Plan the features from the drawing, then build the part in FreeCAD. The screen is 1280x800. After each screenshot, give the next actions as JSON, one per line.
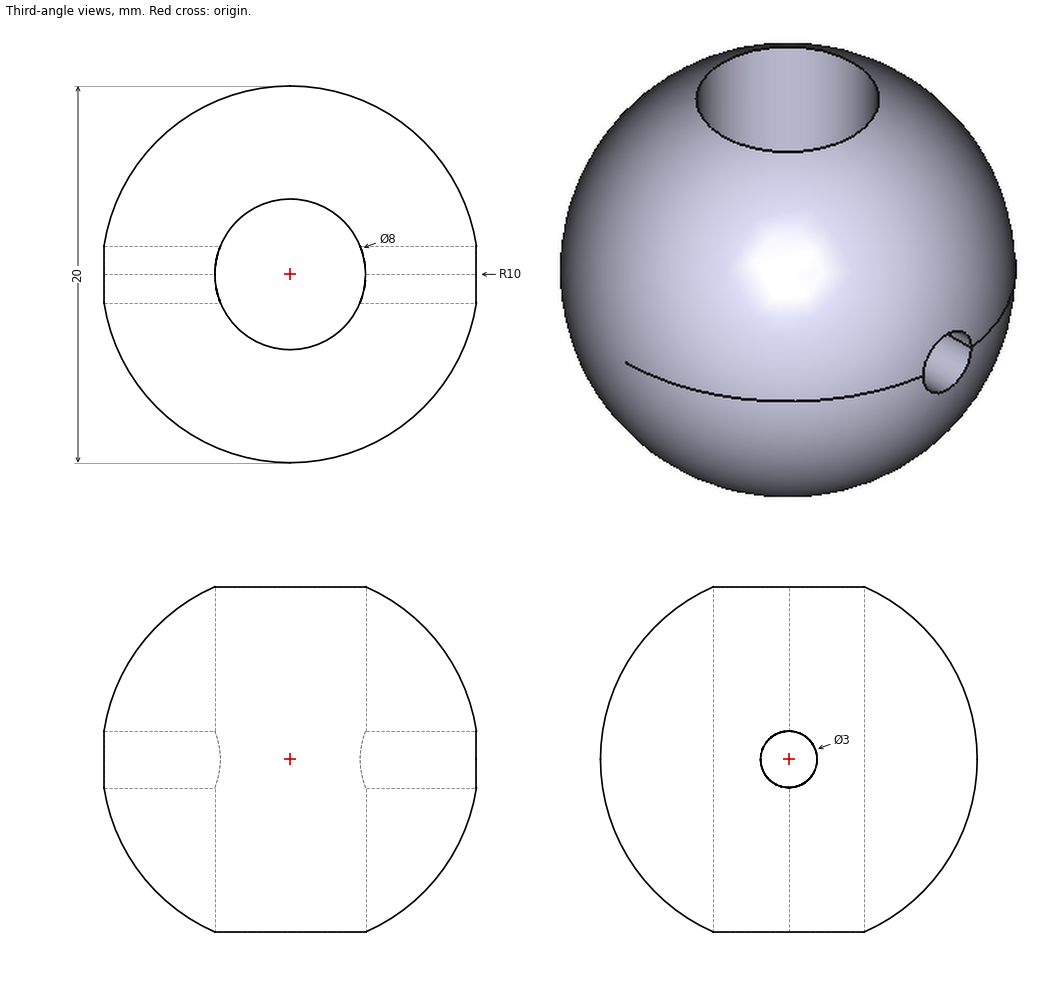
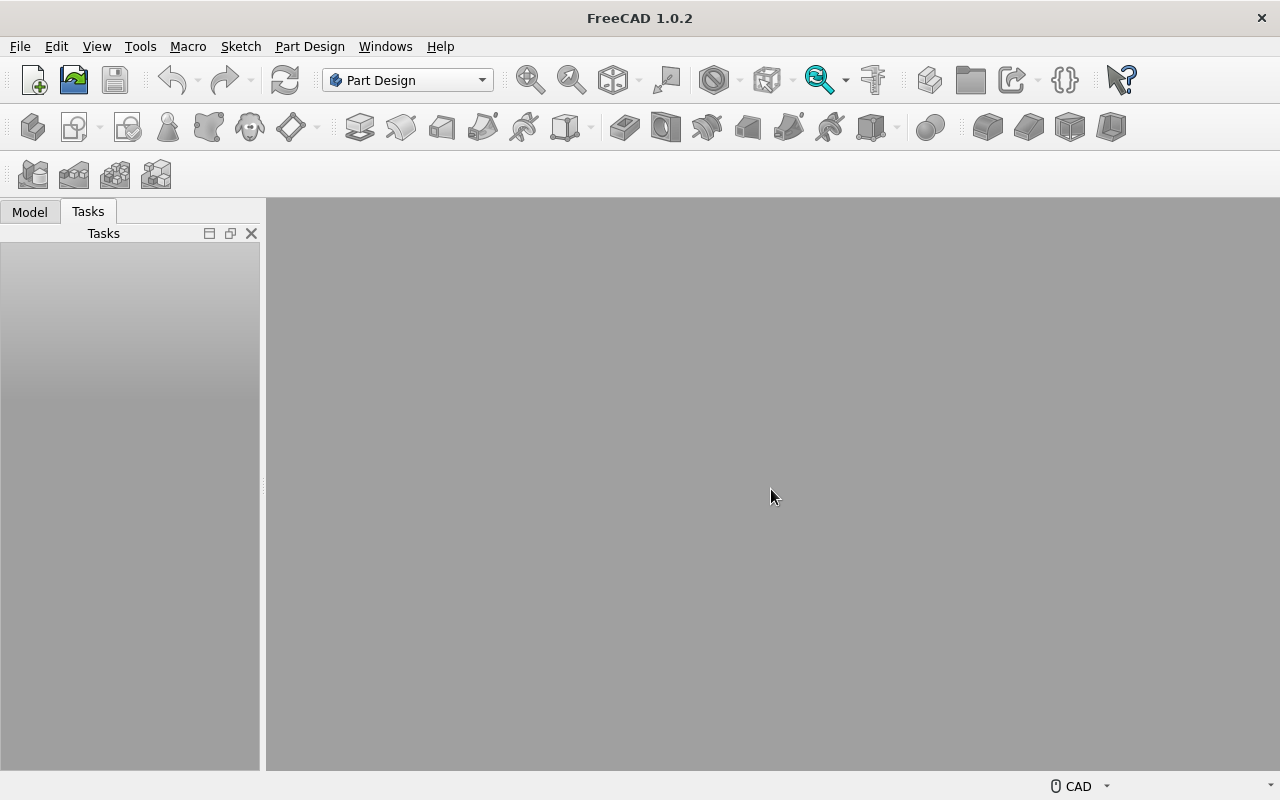
{"action": "left_click", "coordinate": [33, 80]}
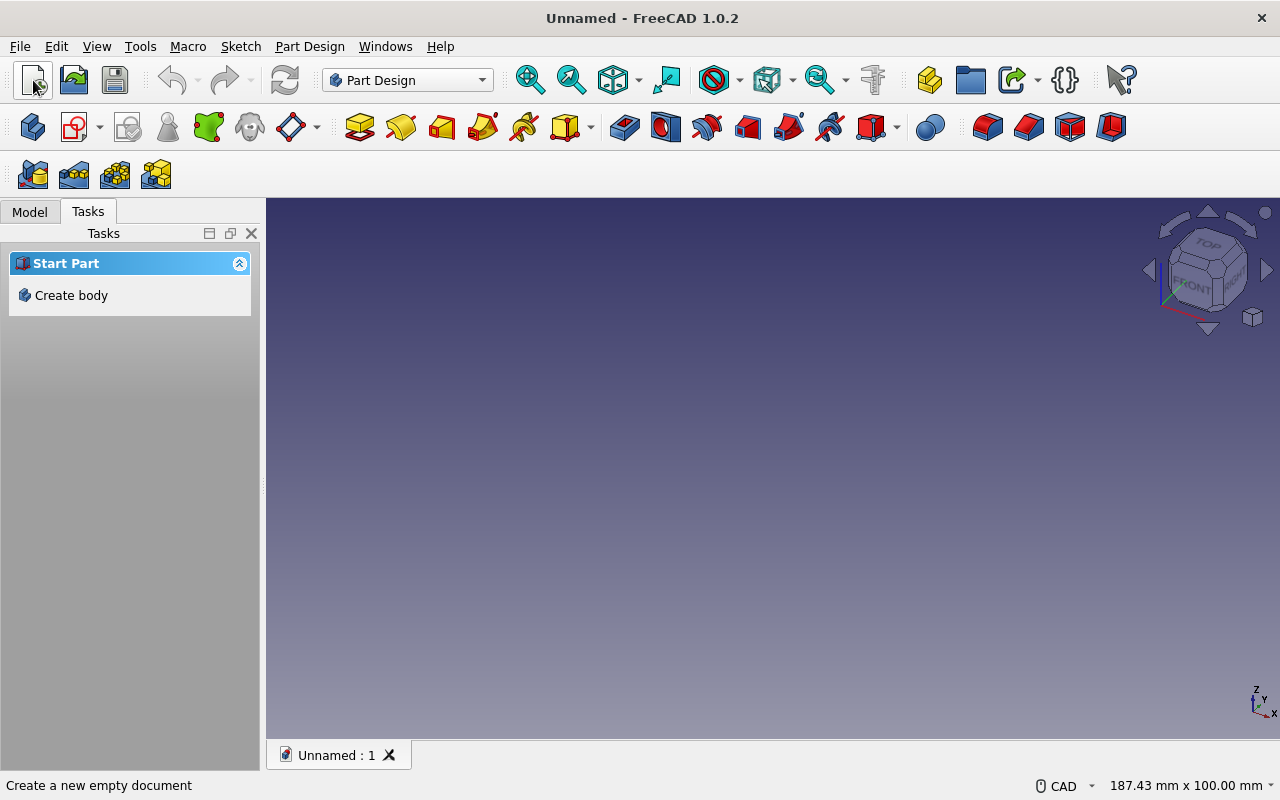
{"action": "left_click", "coordinate": [74, 128]}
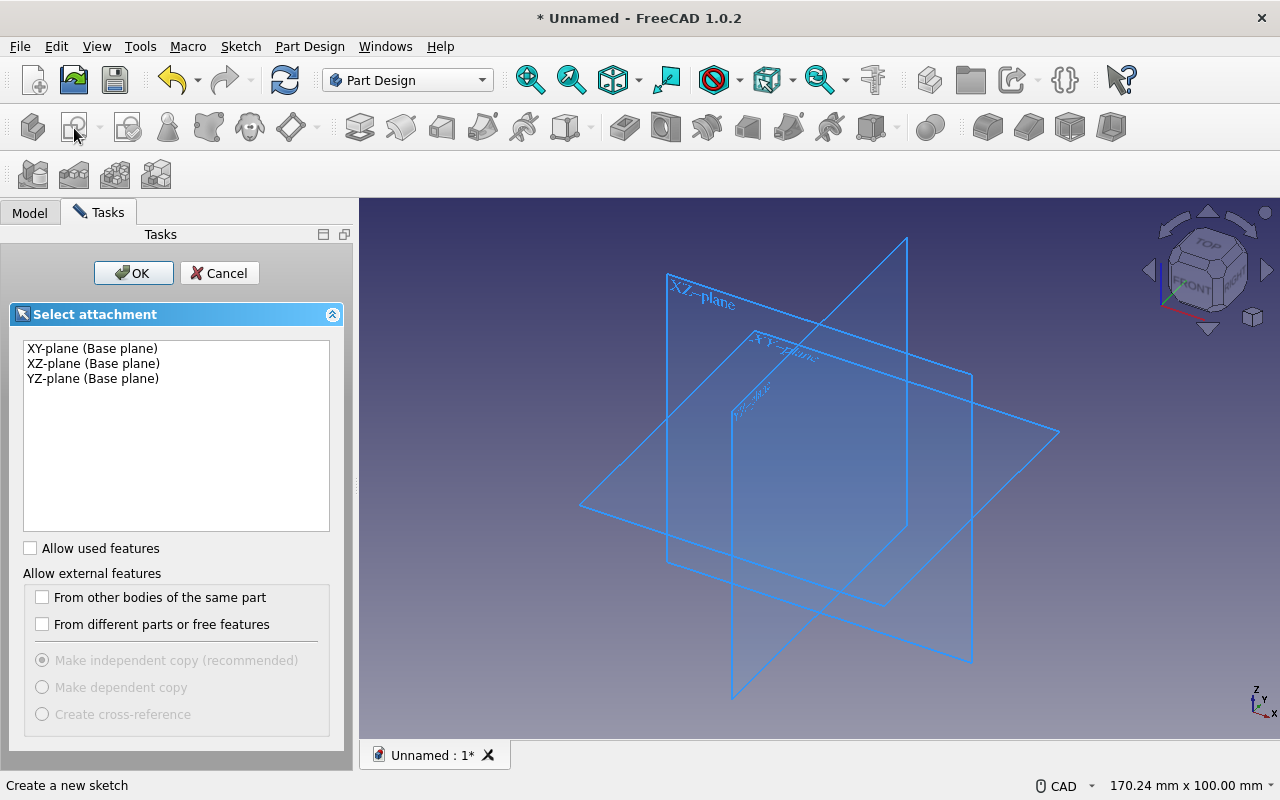
{"action": "left_click", "coordinate": [84, 348]}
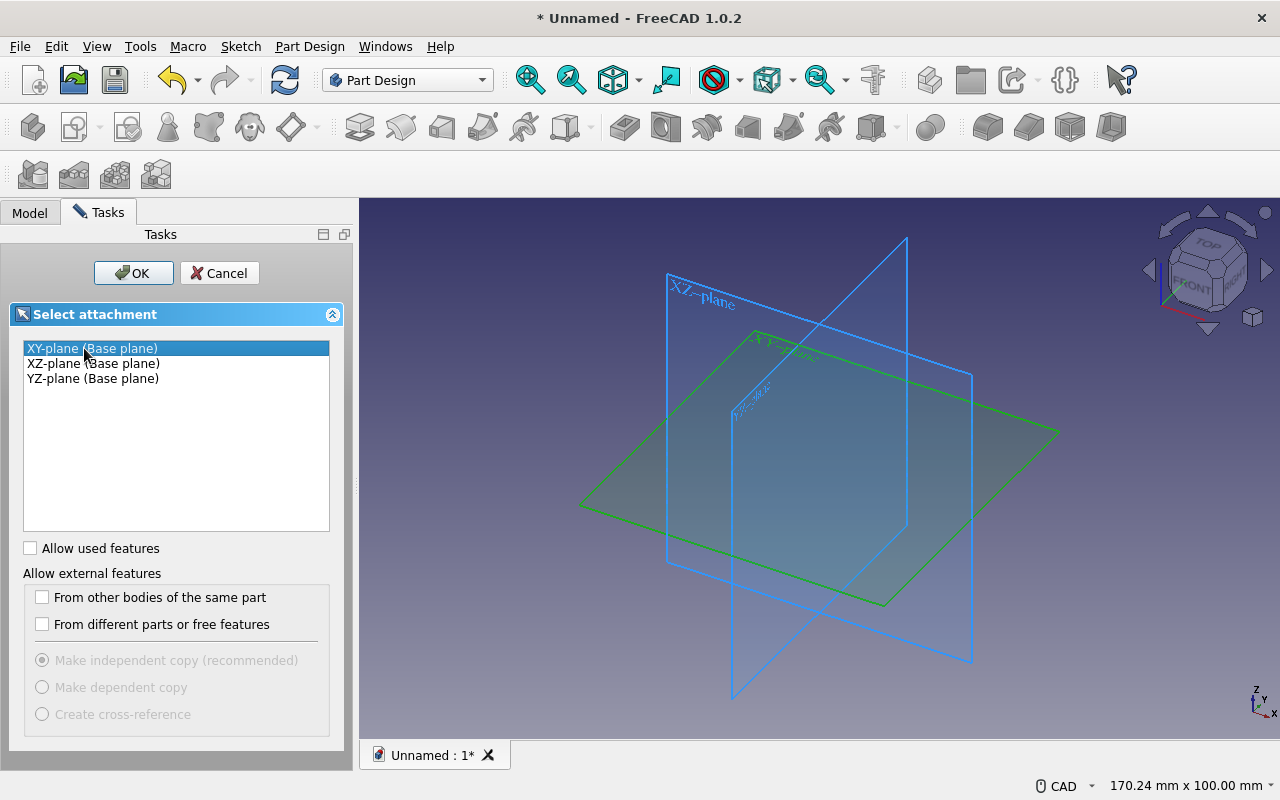
{"action": "left_click", "coordinate": [134, 273]}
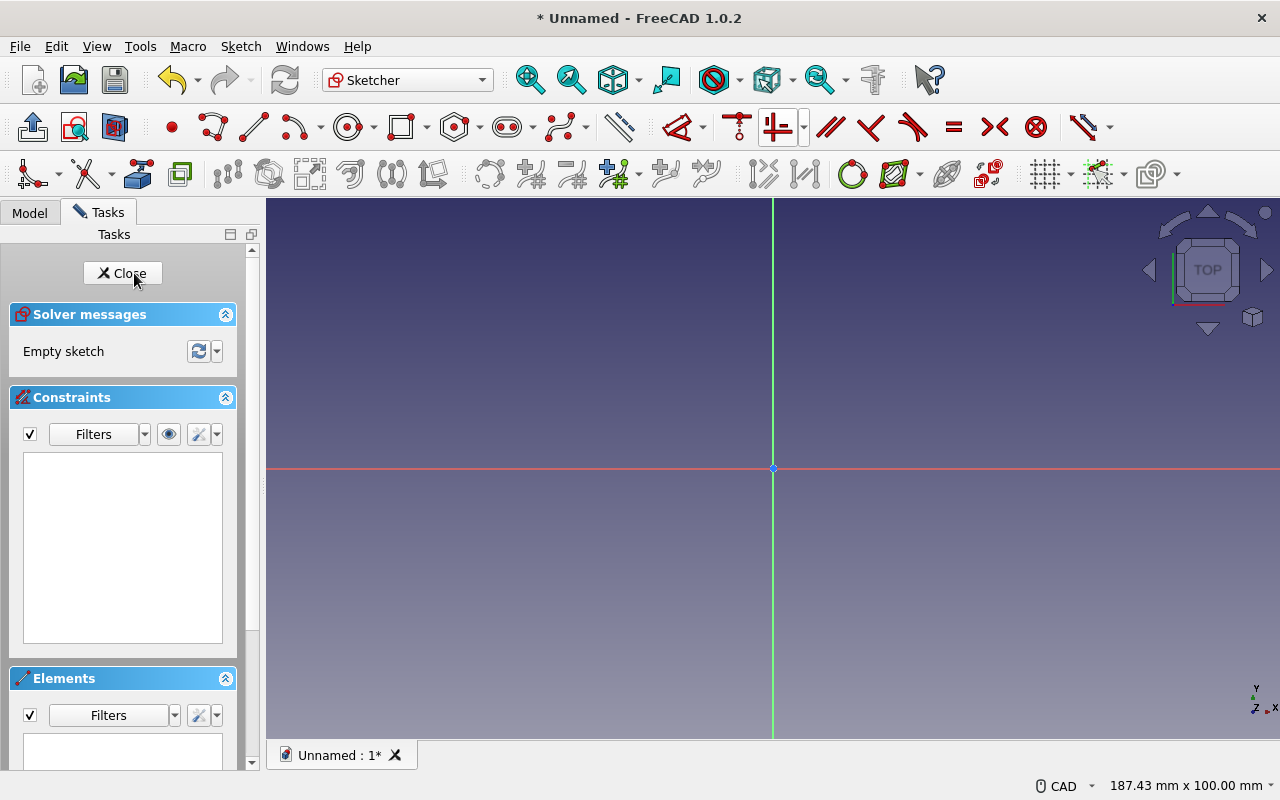
{"action": "scroll", "coordinate": [841, 468], "scroll_direction": "up", "scroll_amount": 6}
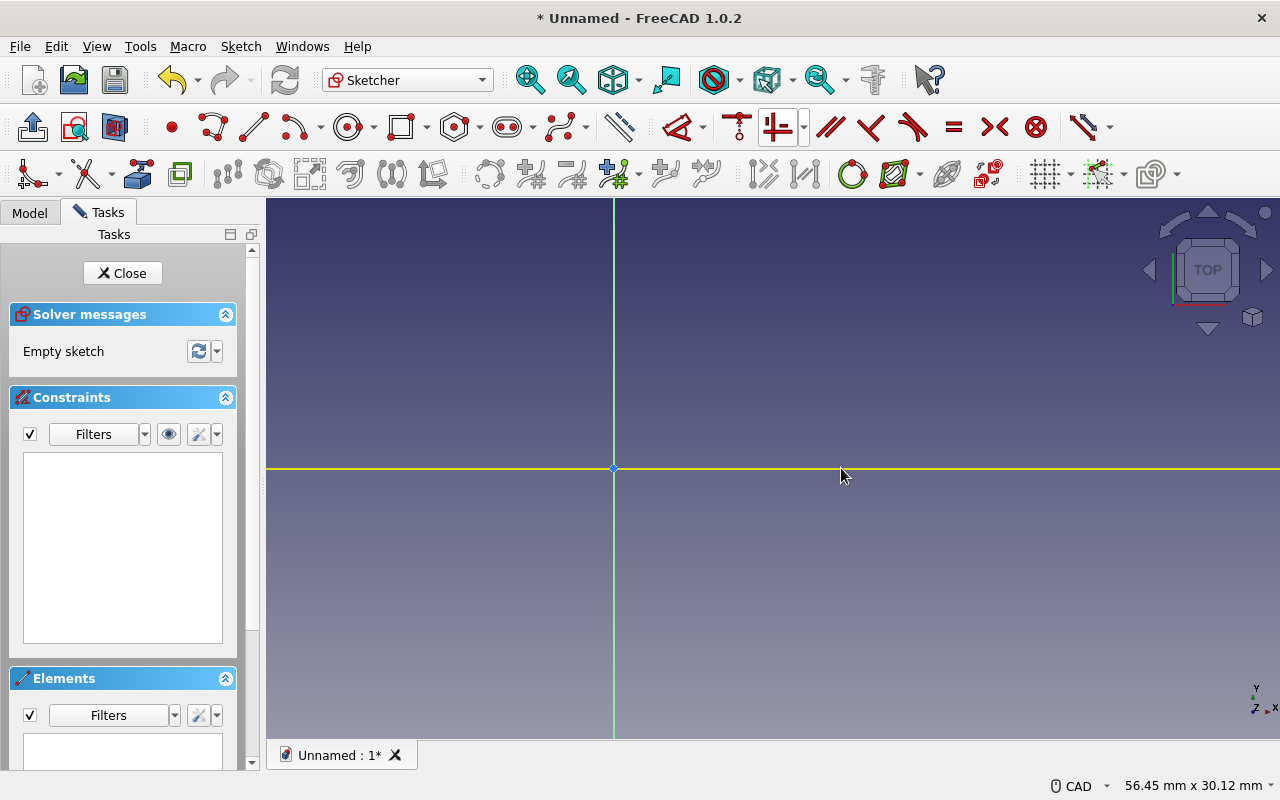
{"action": "left_click", "coordinate": [254, 128]}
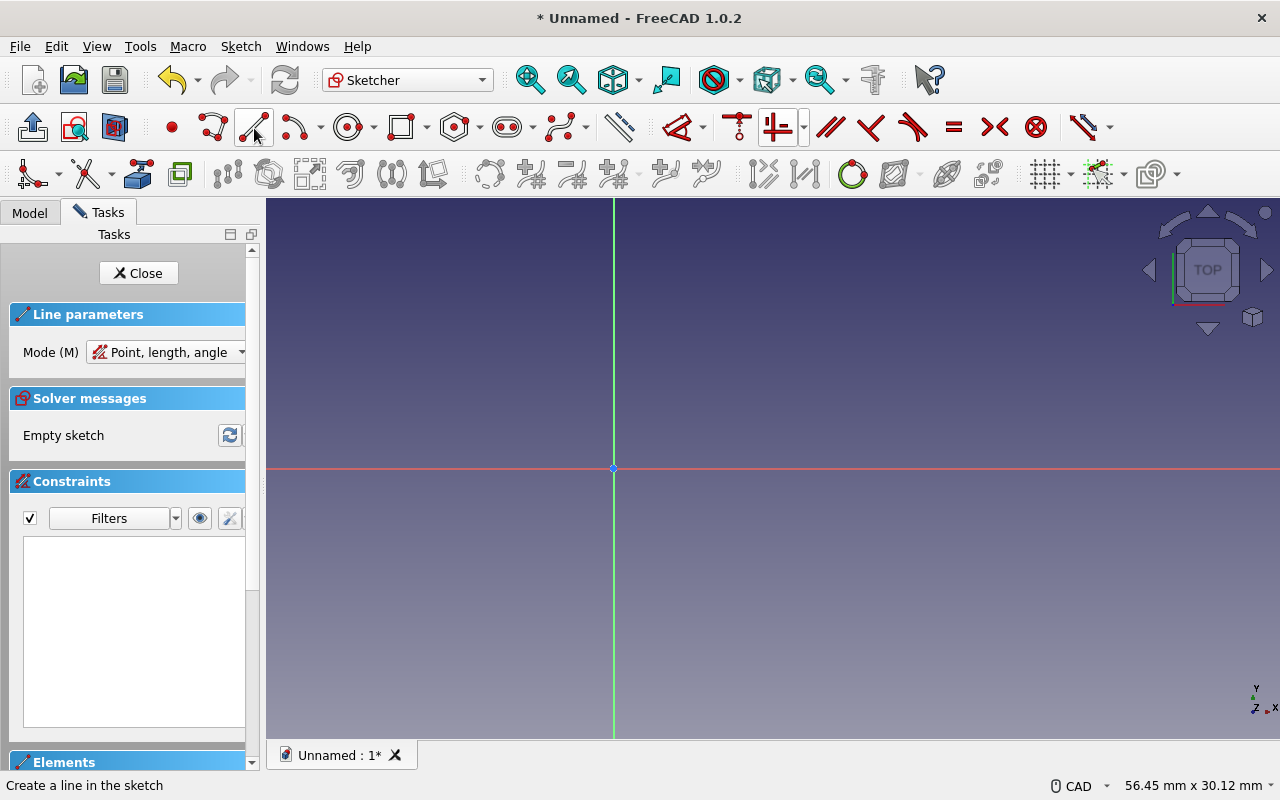
{"action": "left_click", "coordinate": [614, 289]}
{"action": "left_click", "coordinate": [623, 648]}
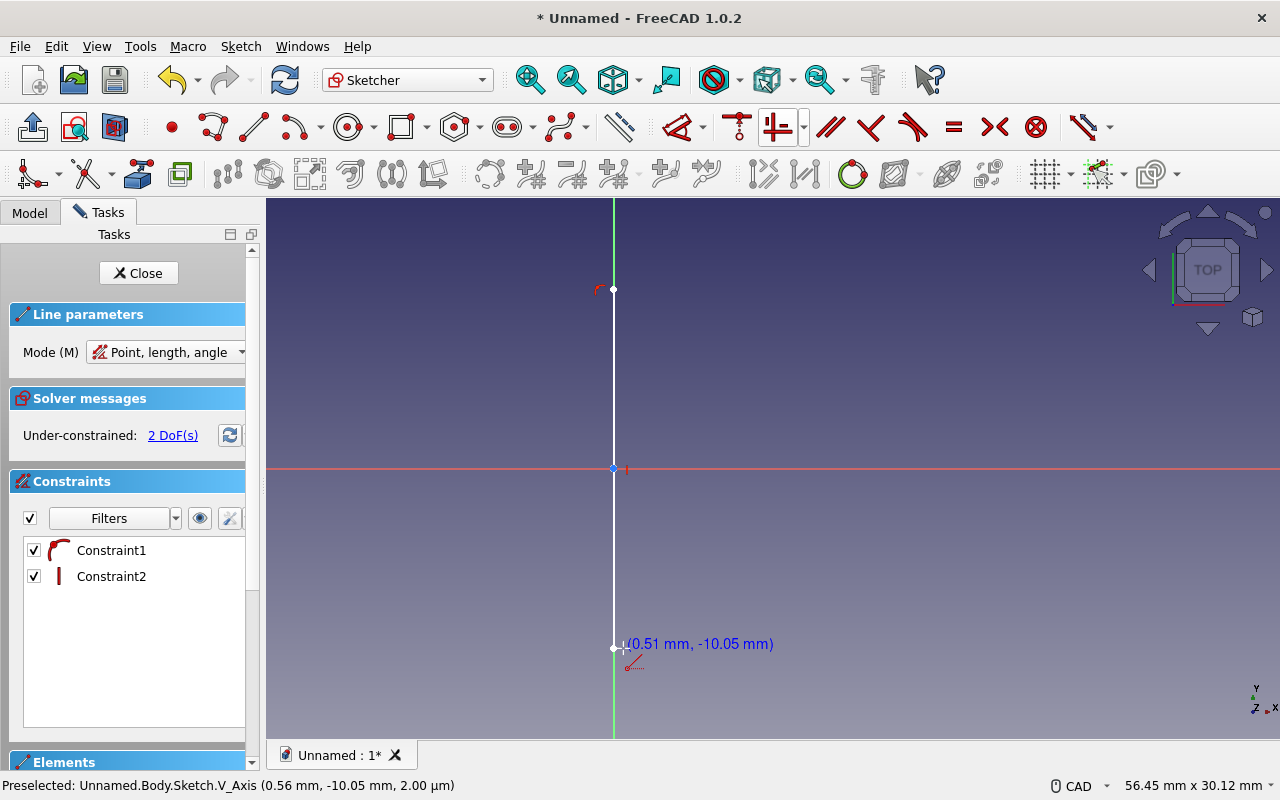
{"action": "key", "text": "g 3 a"}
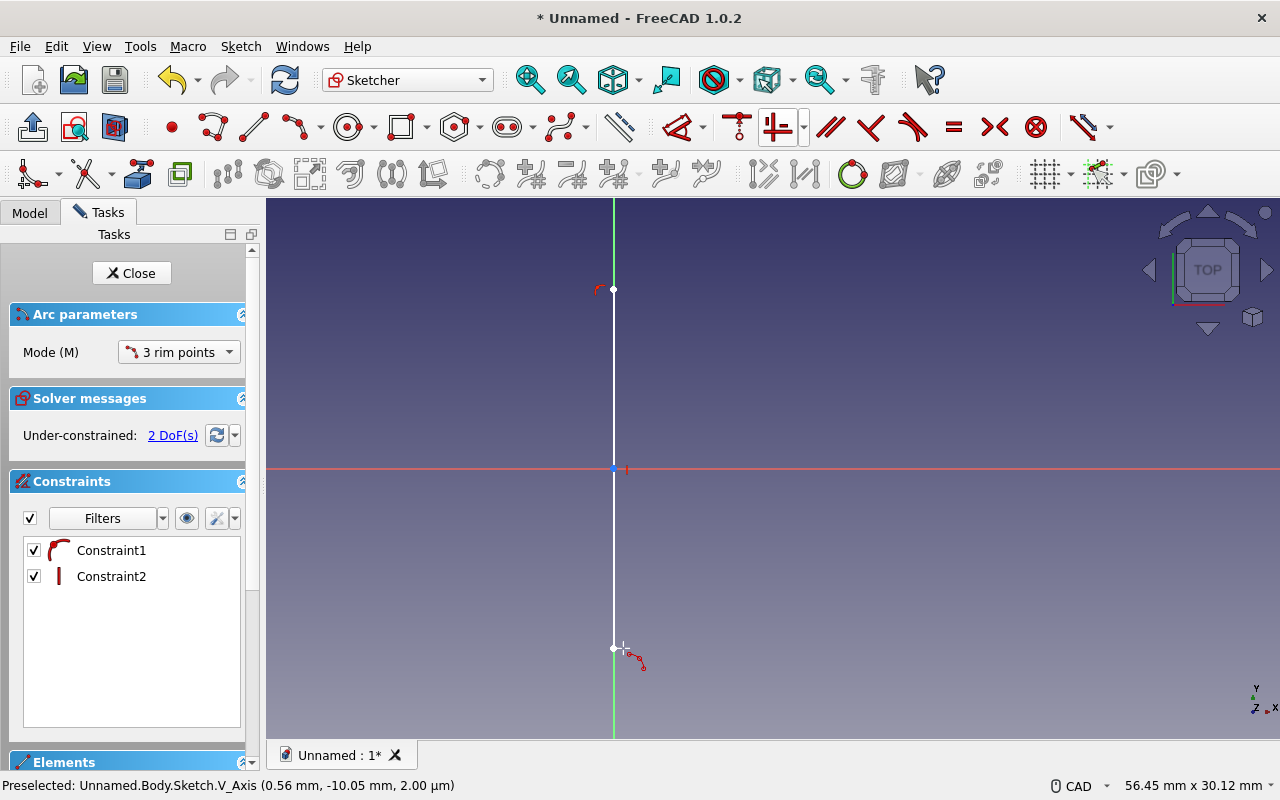
{"action": "left_click", "coordinate": [623, 648]}
{"action": "left_click", "coordinate": [614, 290]}
{"action": "left_click", "coordinate": [785, 524]}
{"action": "key", "text": "Escape"}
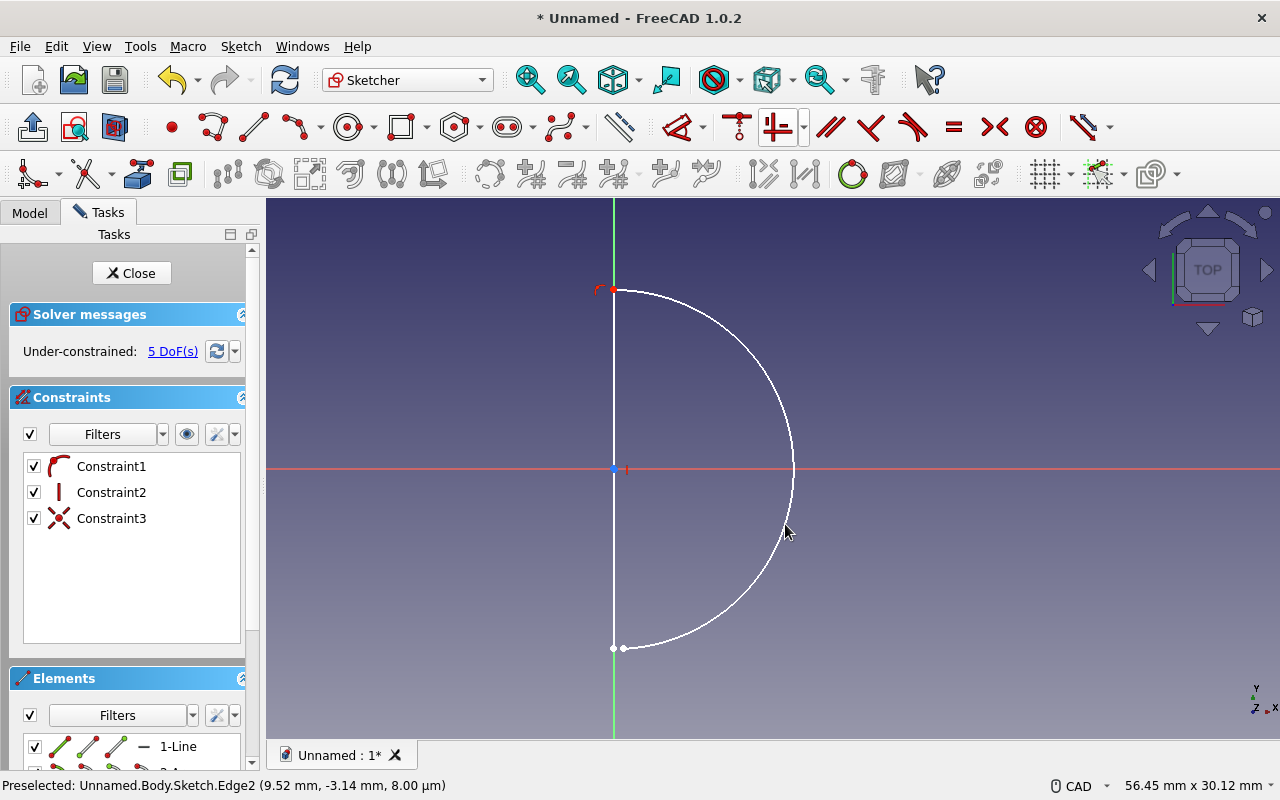
{"action": "left_click_drag", "start_coordinate": [604, 458], "coordinate": [624, 480]}